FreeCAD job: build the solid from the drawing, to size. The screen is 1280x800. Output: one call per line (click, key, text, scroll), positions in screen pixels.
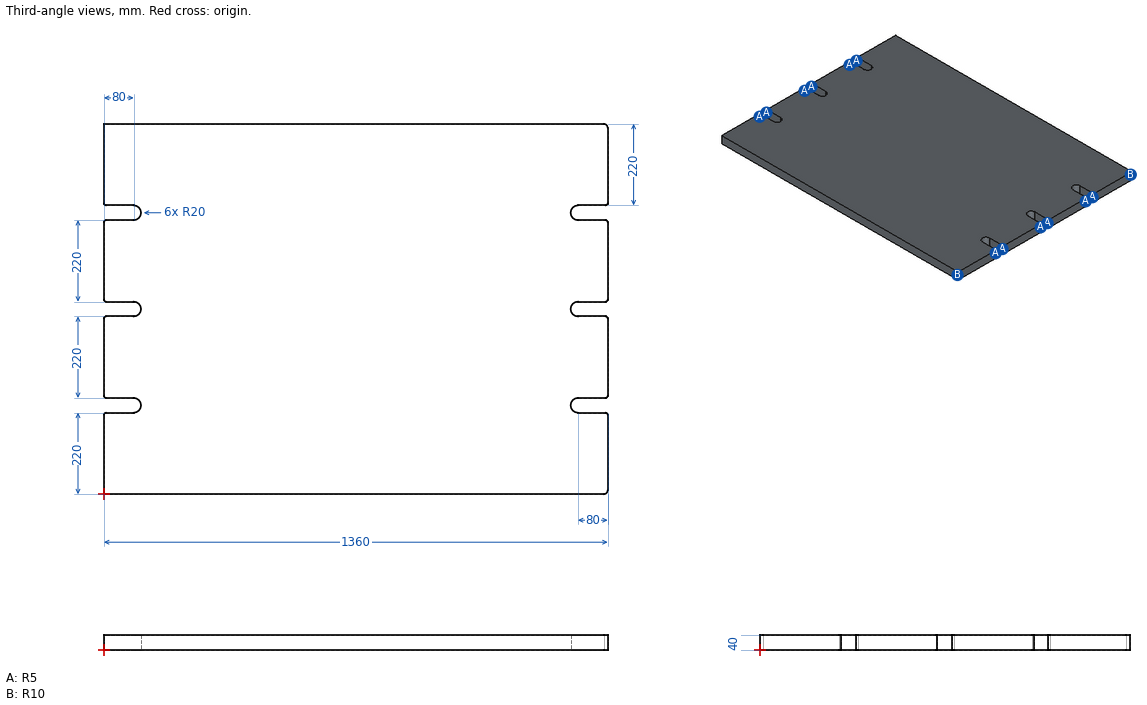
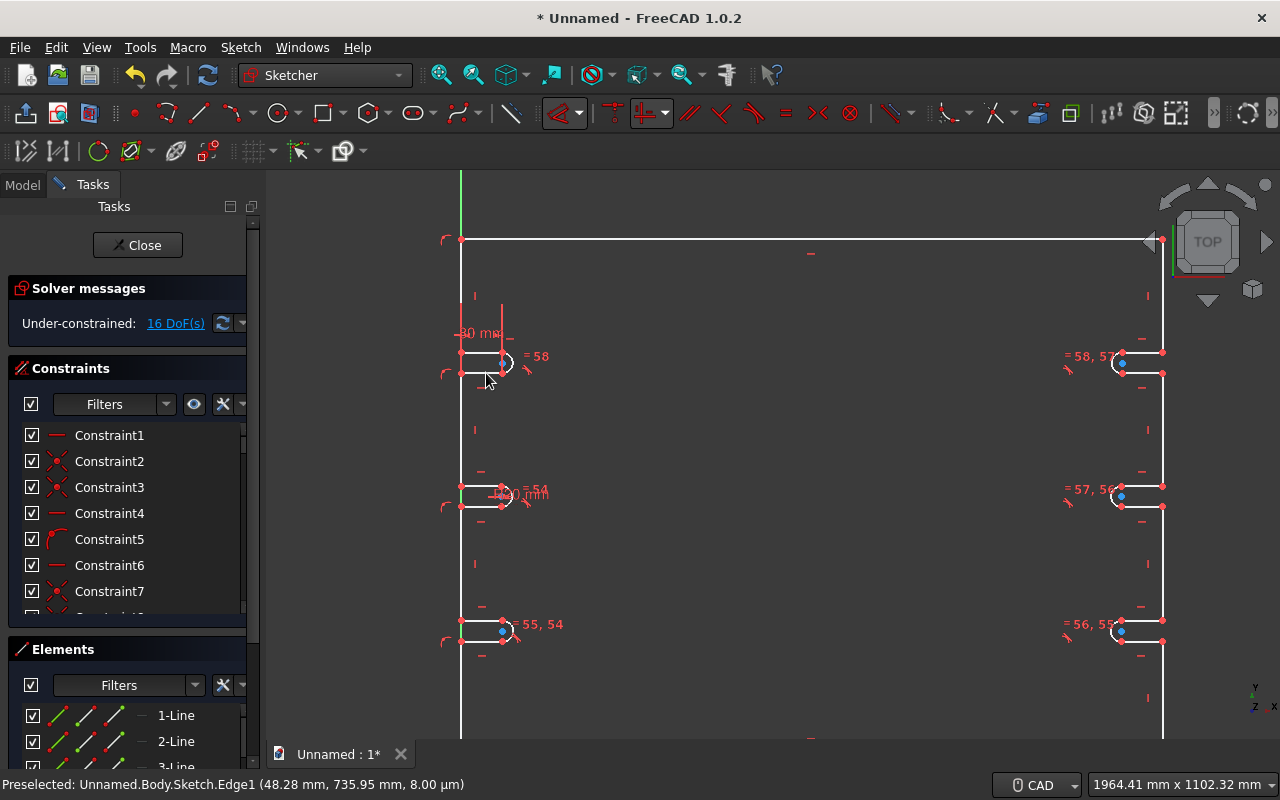
click(473, 486)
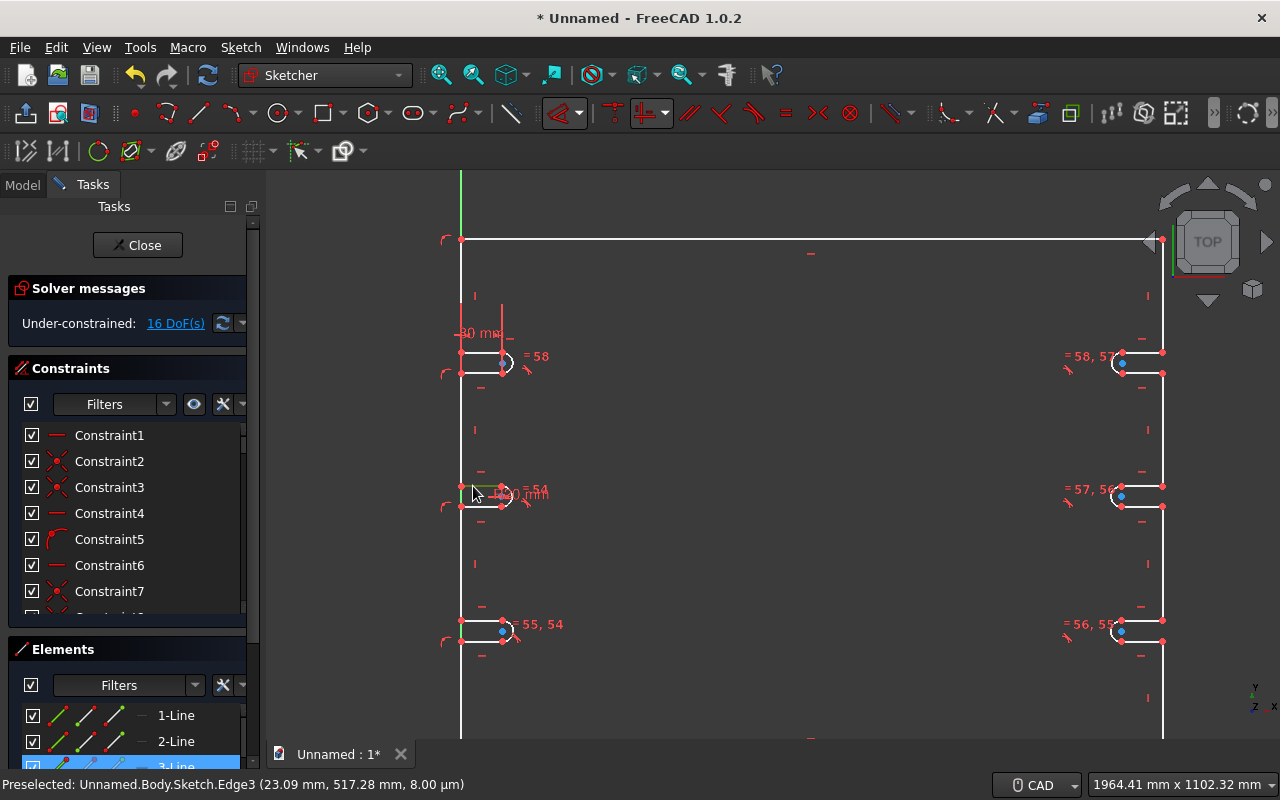
click(582, 114)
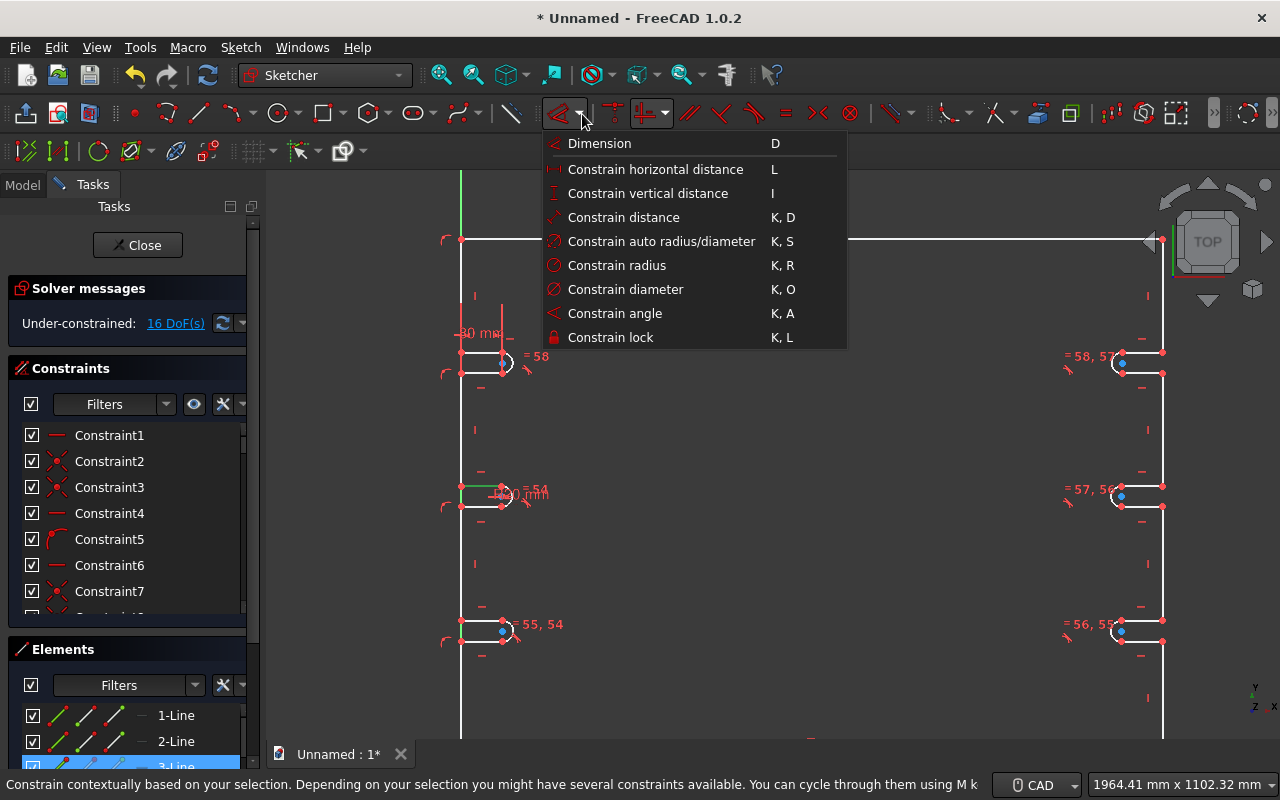
click(695, 169)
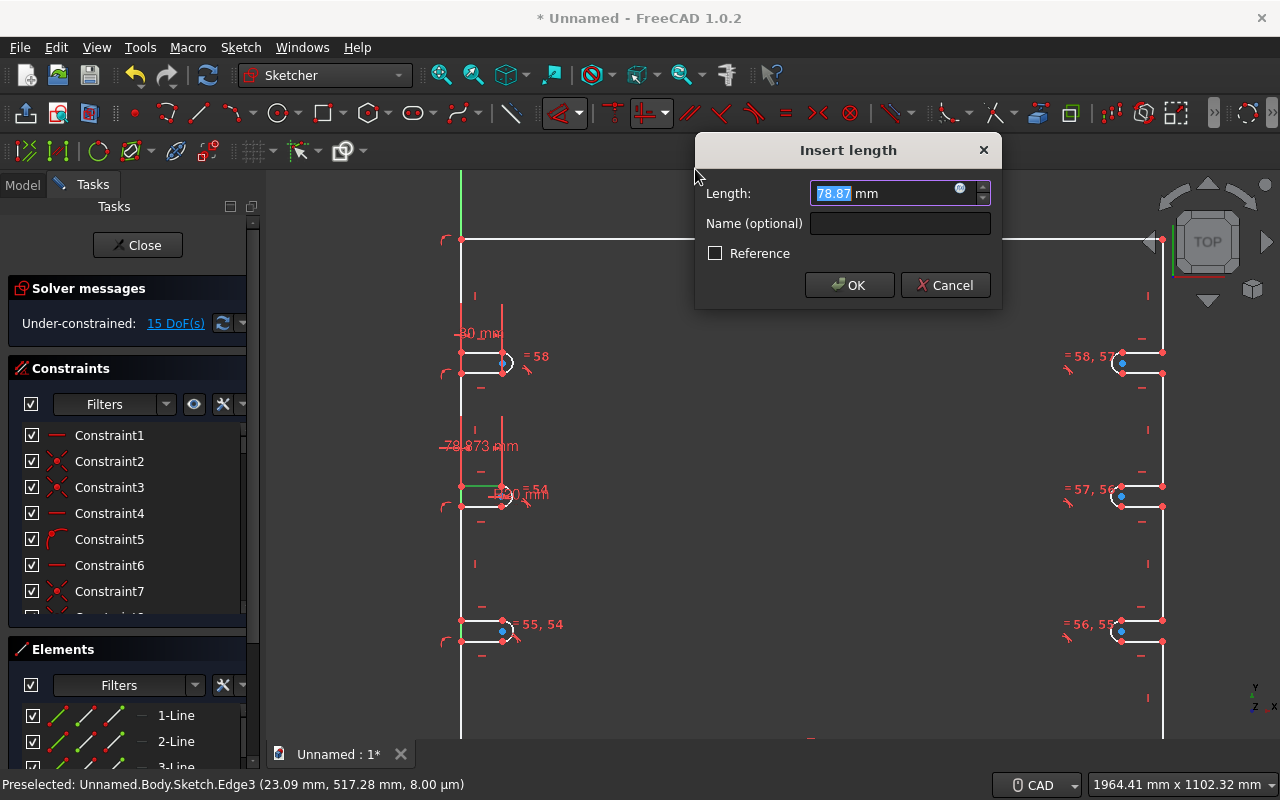
text(80)
key(Return)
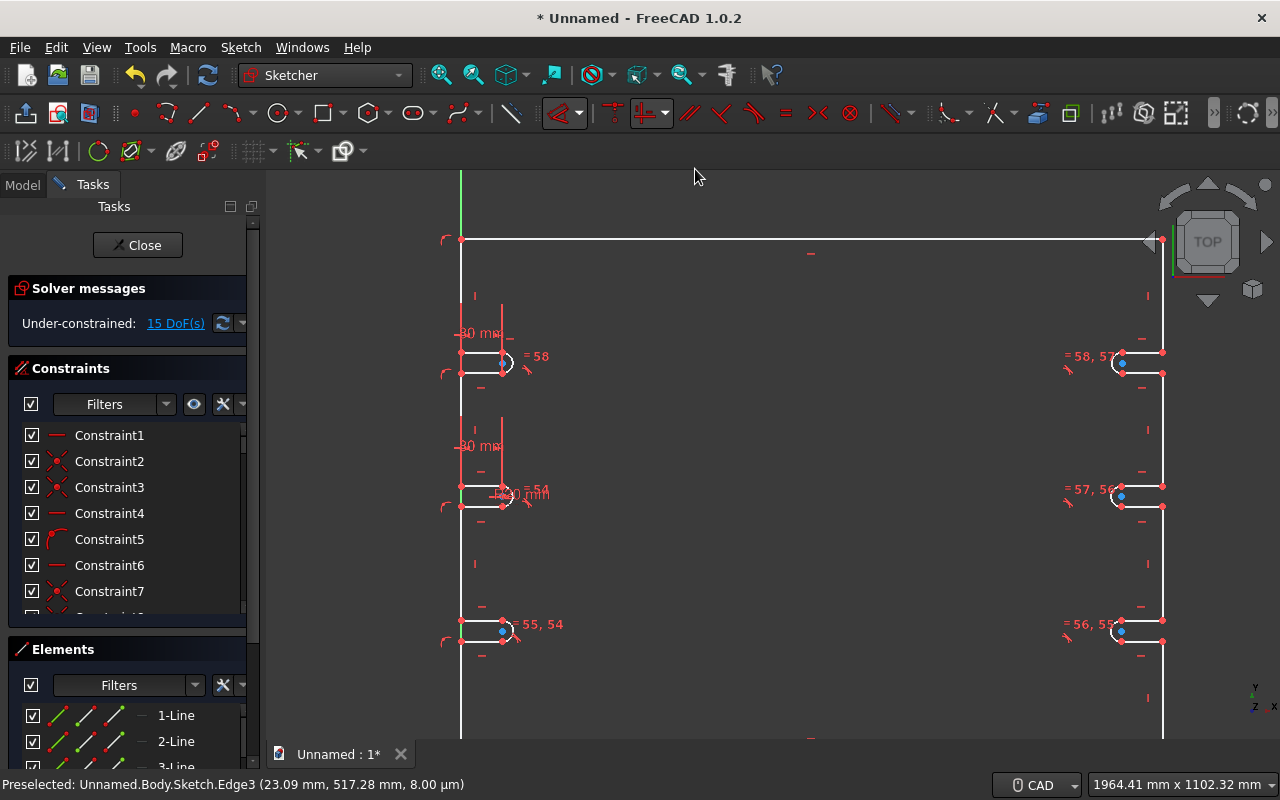
click(474, 621)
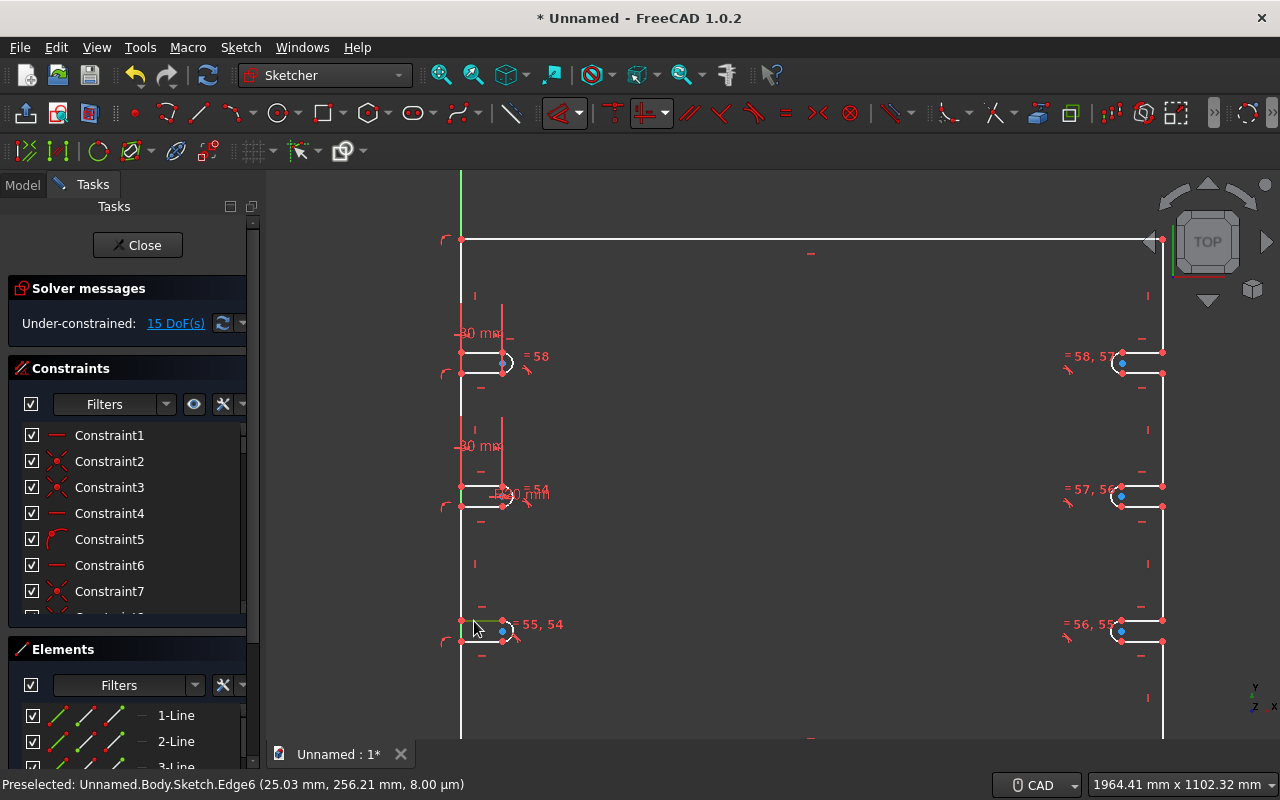
click(582, 114)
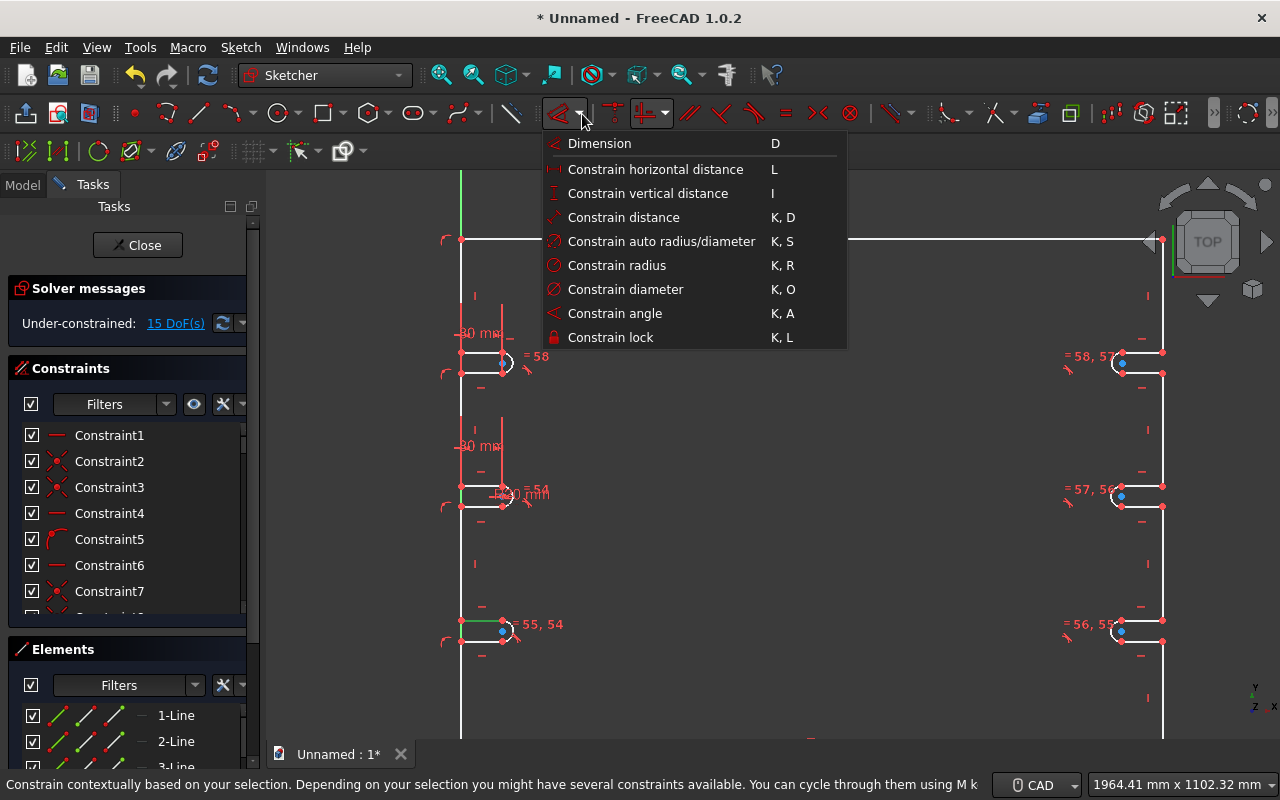
click(695, 169)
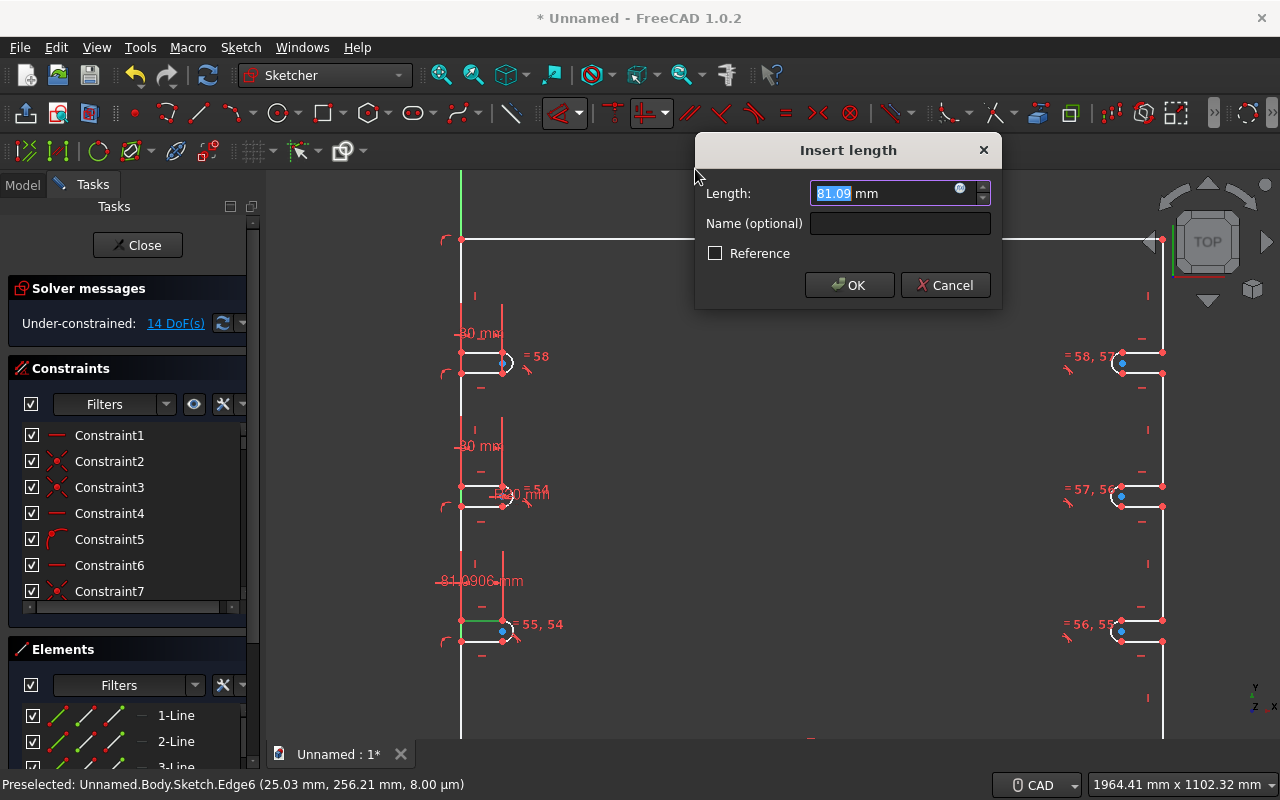
text(80)
key(Return)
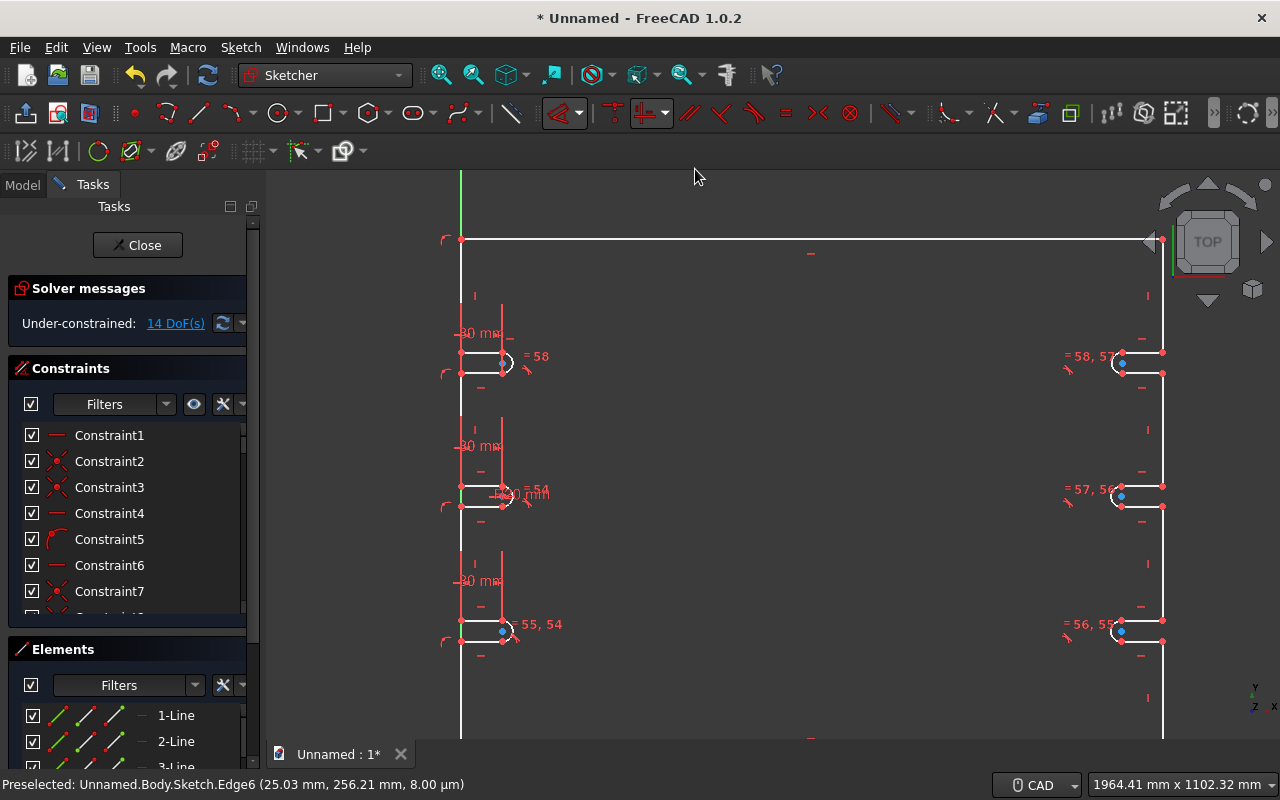
scroll(486, 372, down, 2)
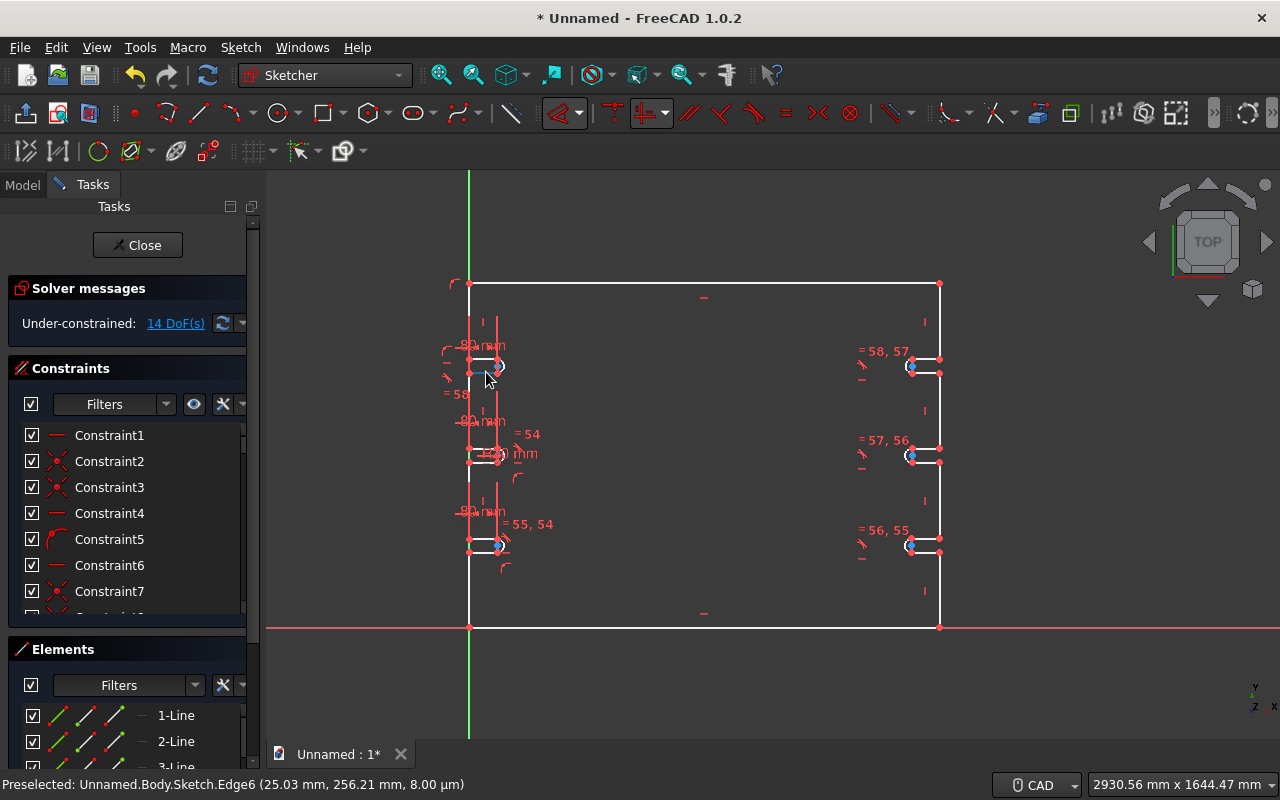
scroll(931, 553, up, 3)